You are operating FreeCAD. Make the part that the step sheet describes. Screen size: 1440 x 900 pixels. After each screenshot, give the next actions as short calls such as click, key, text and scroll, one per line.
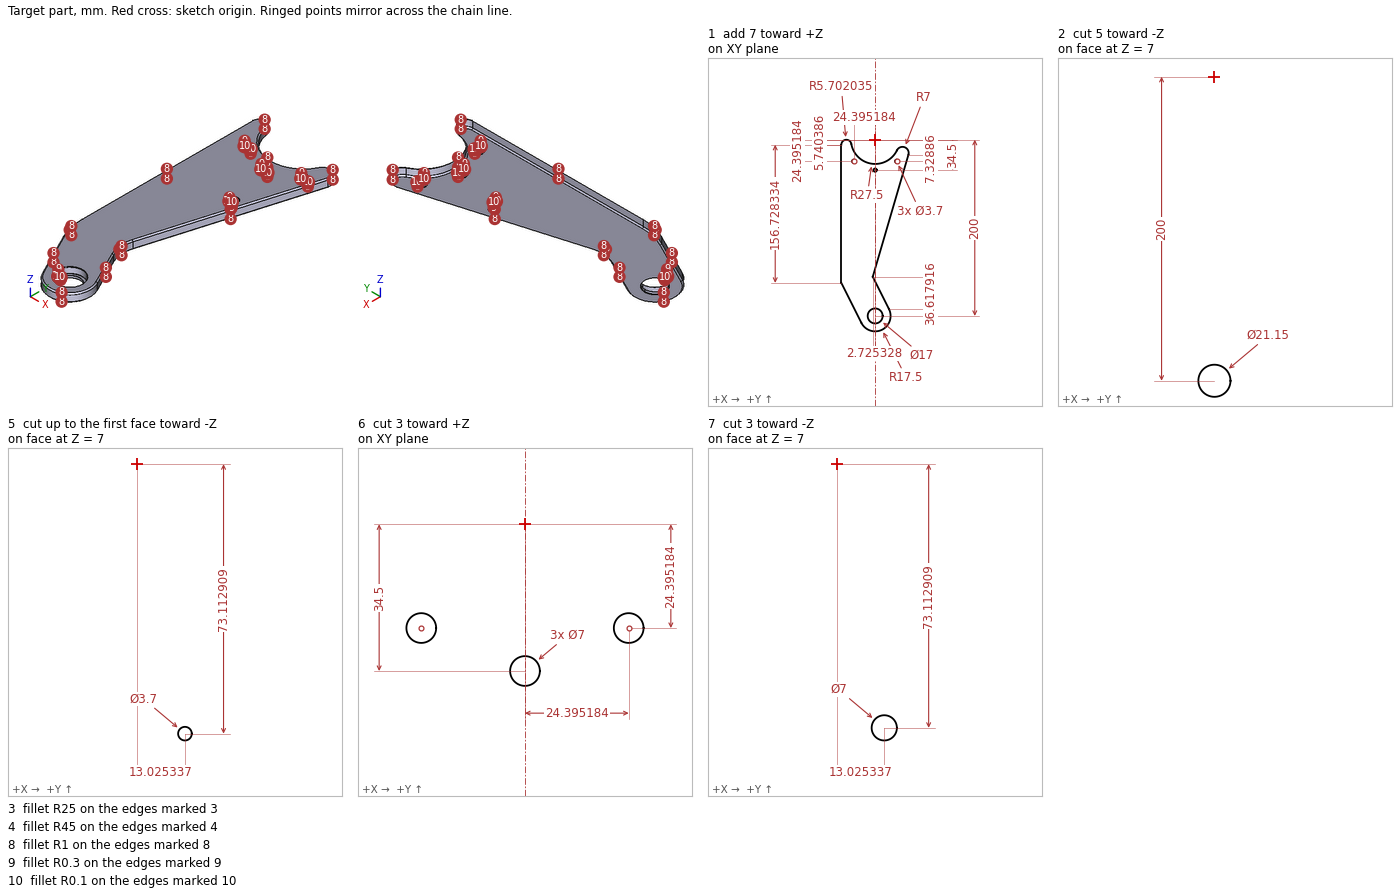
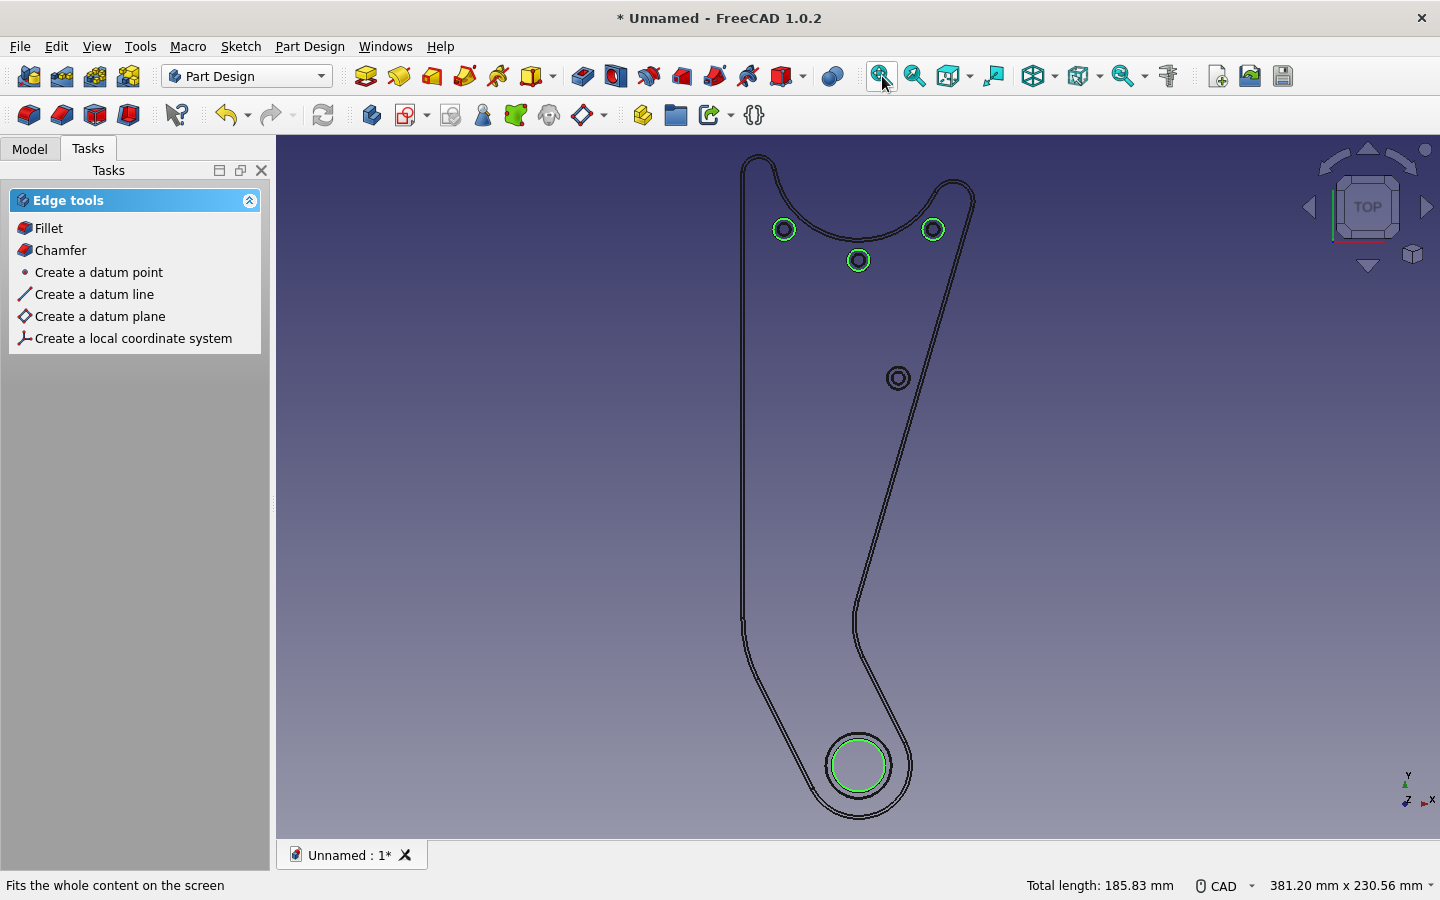
scroll(853, 259, up, 6)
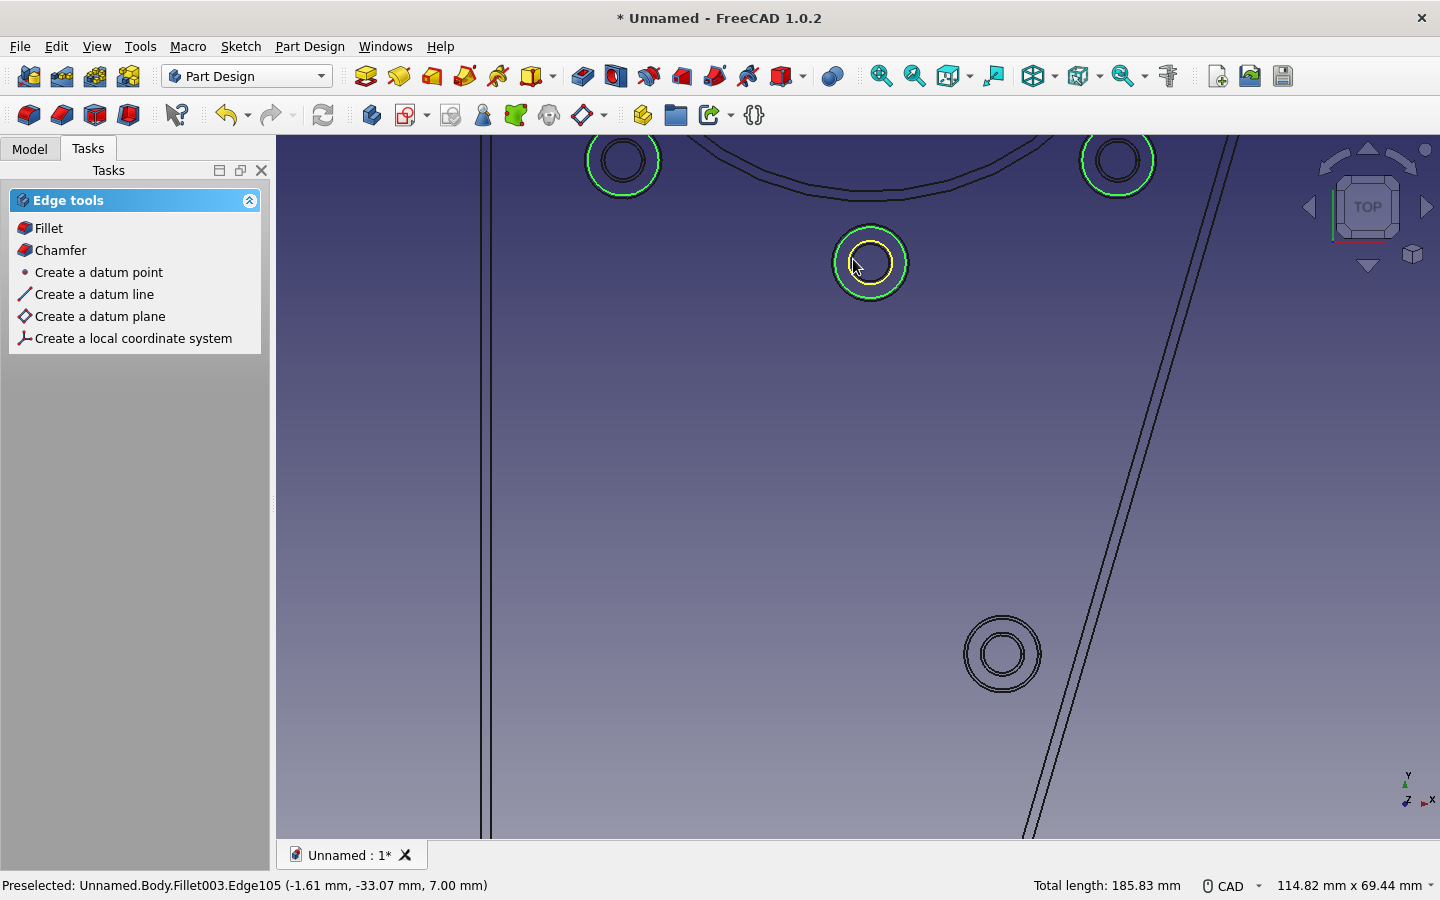
click(984, 653, ctrl)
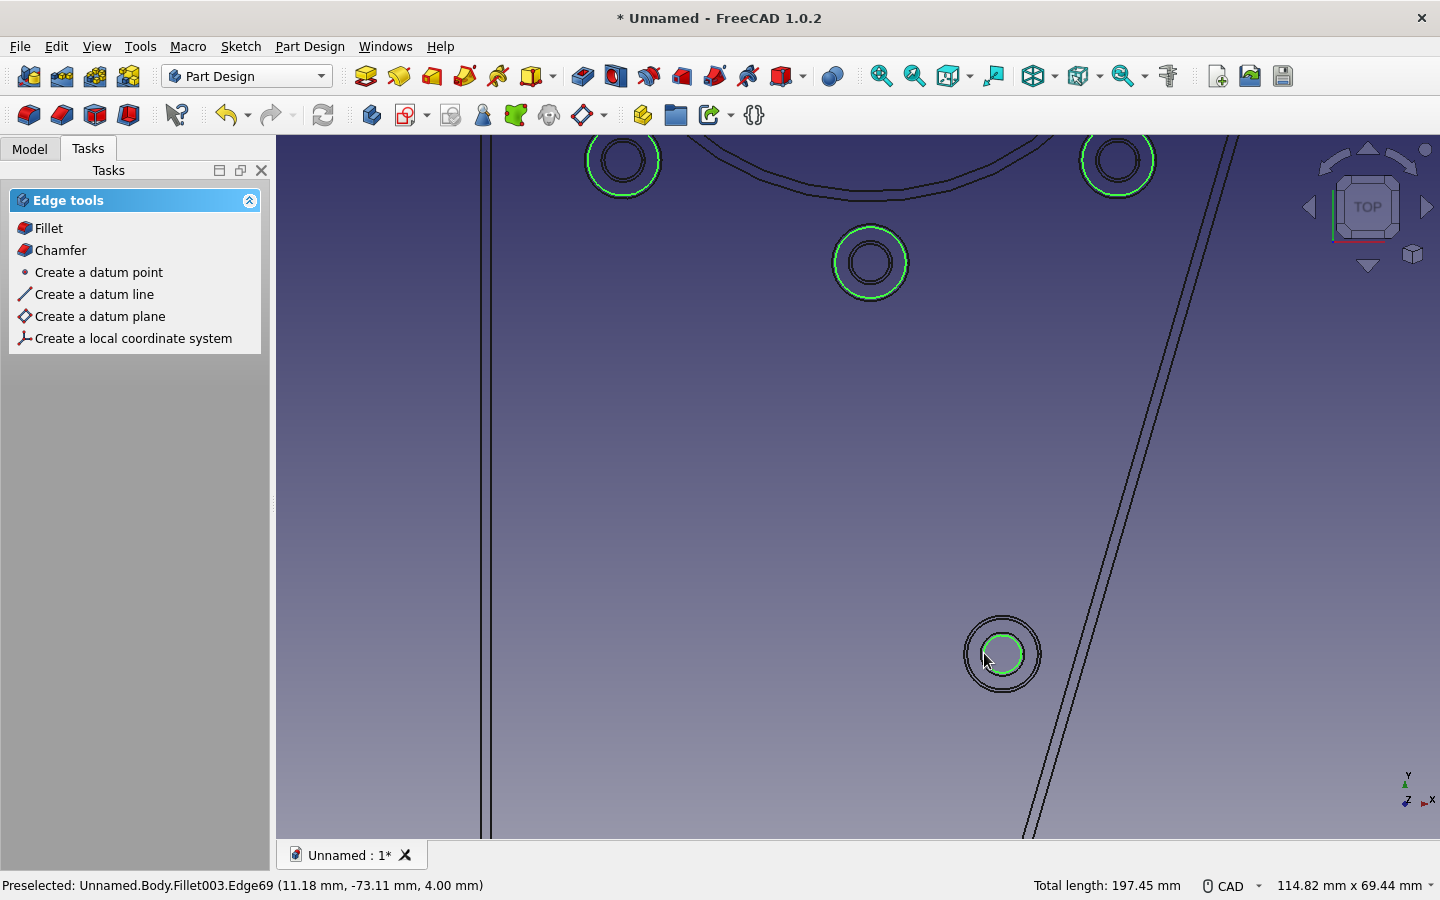
click(882, 76)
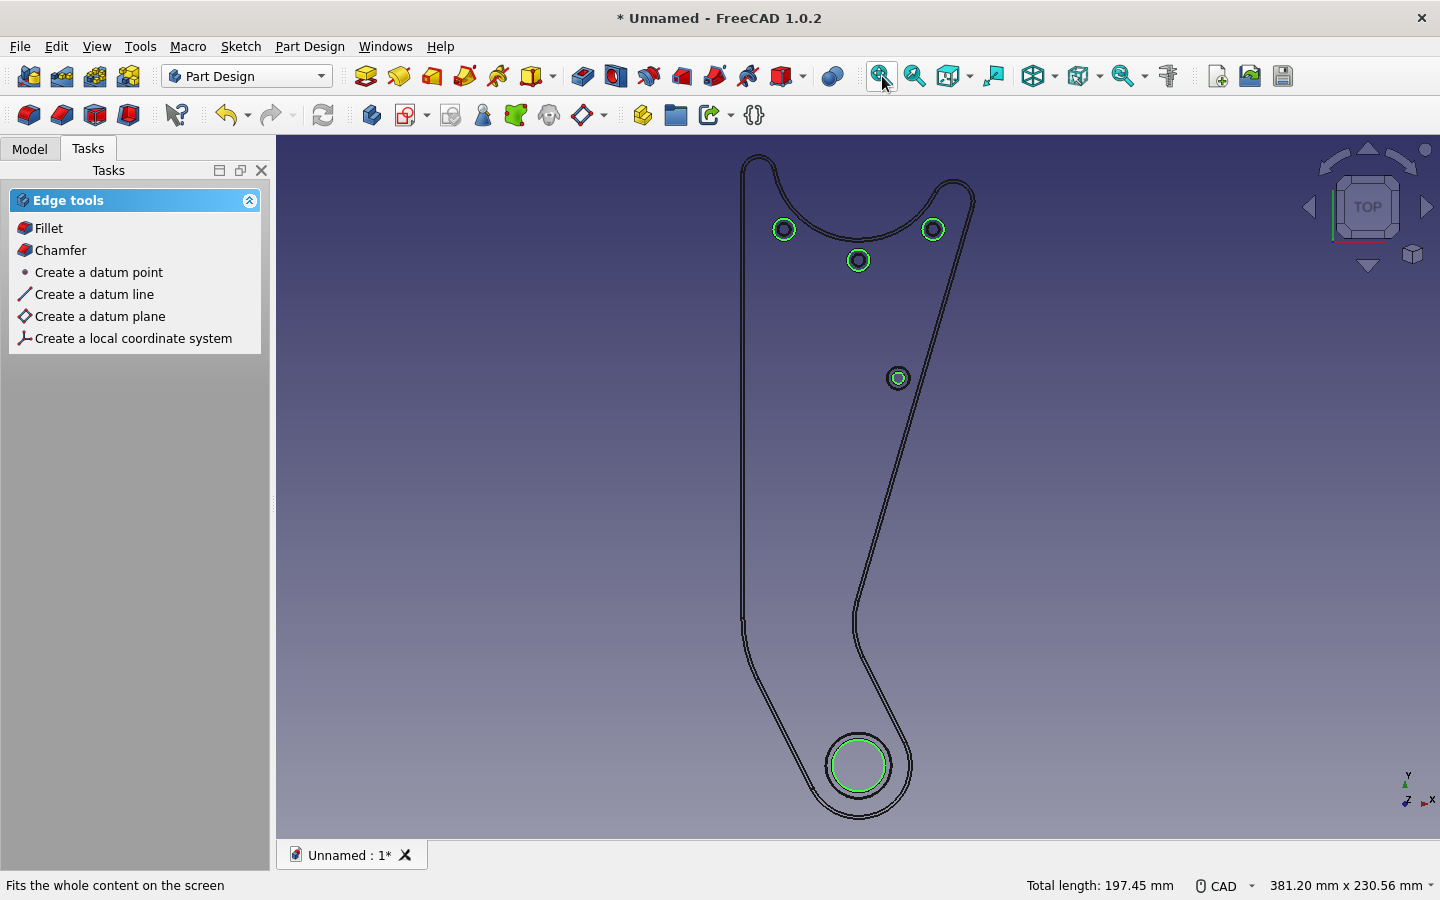
key(1)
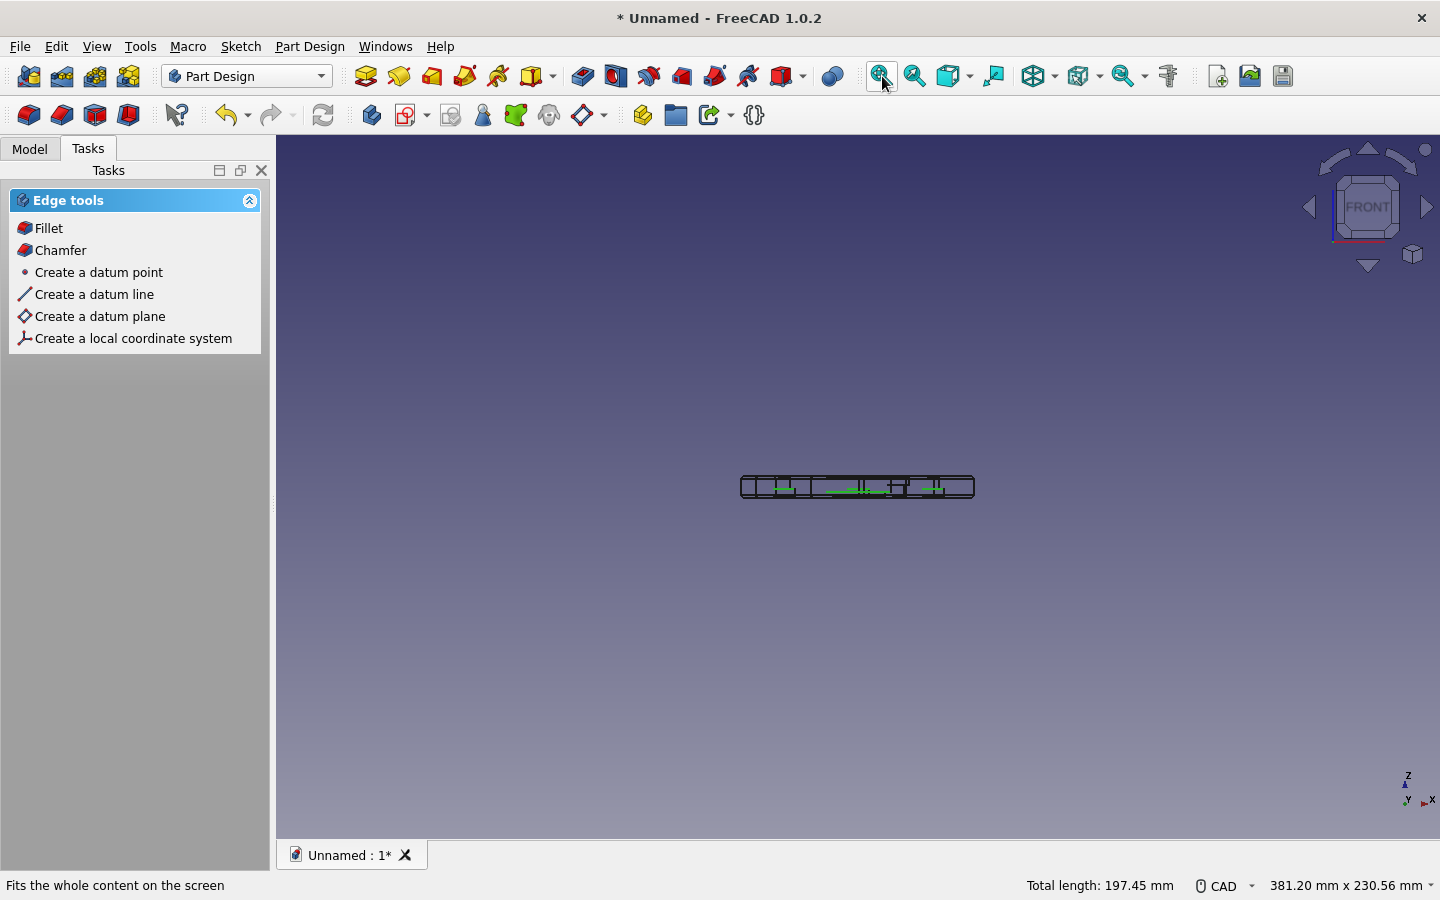
click(882, 76)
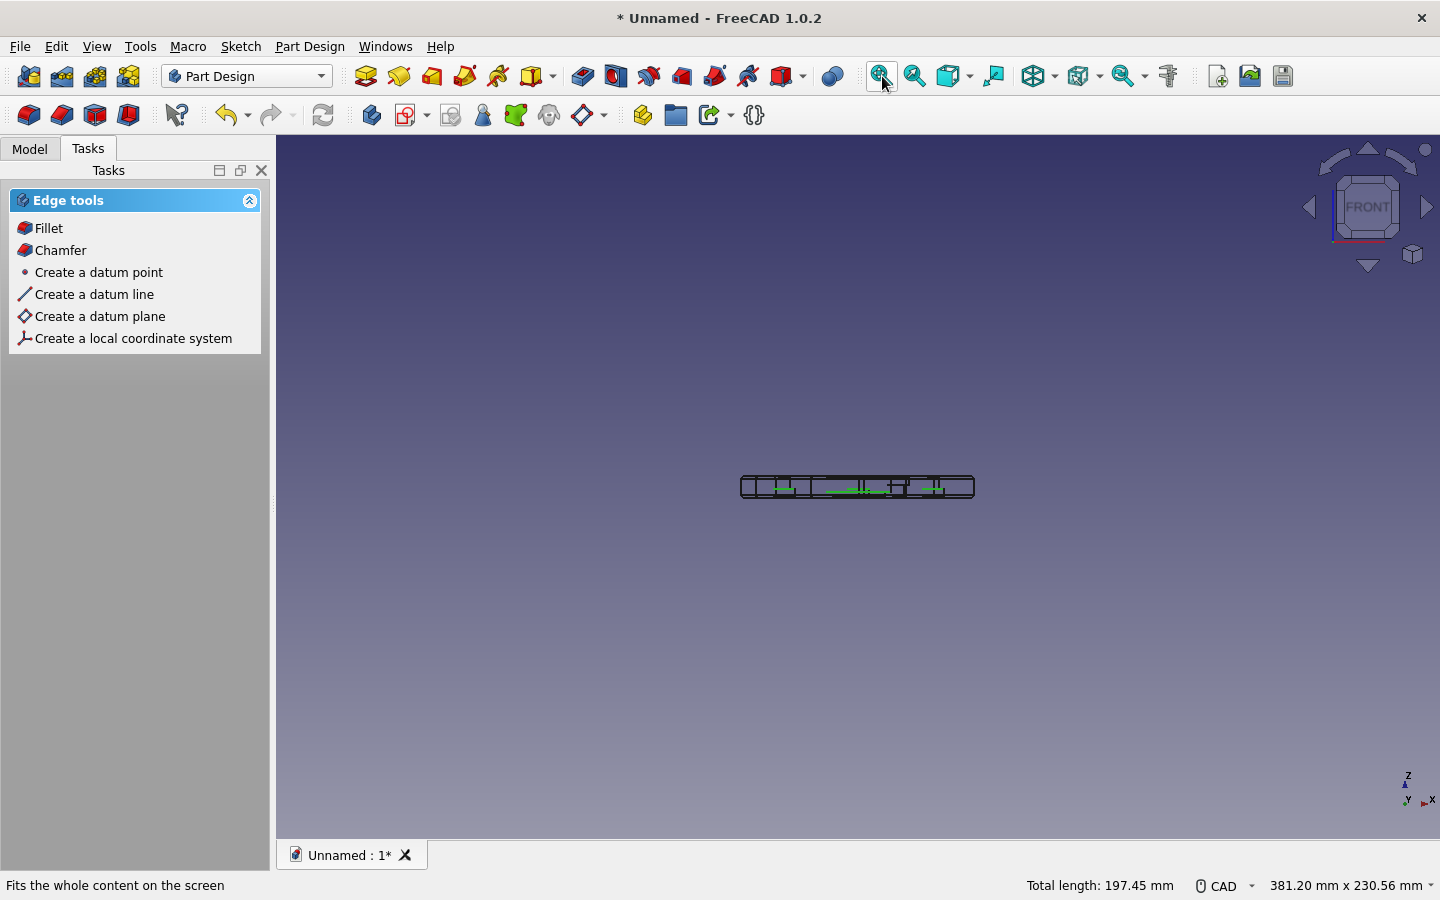
scroll(853, 488, up, 6)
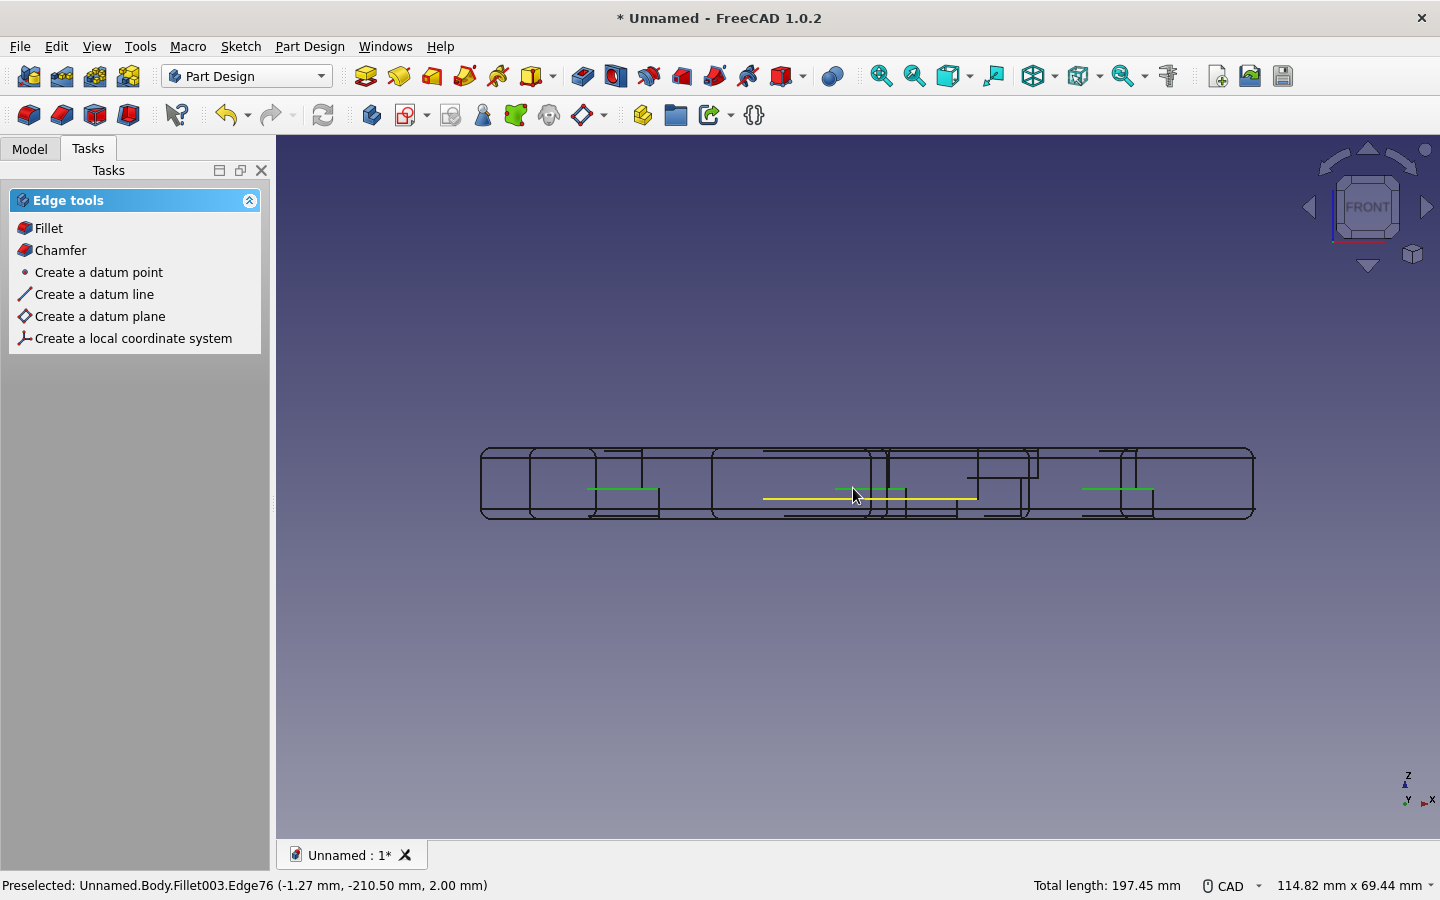
click(992, 477, ctrl)